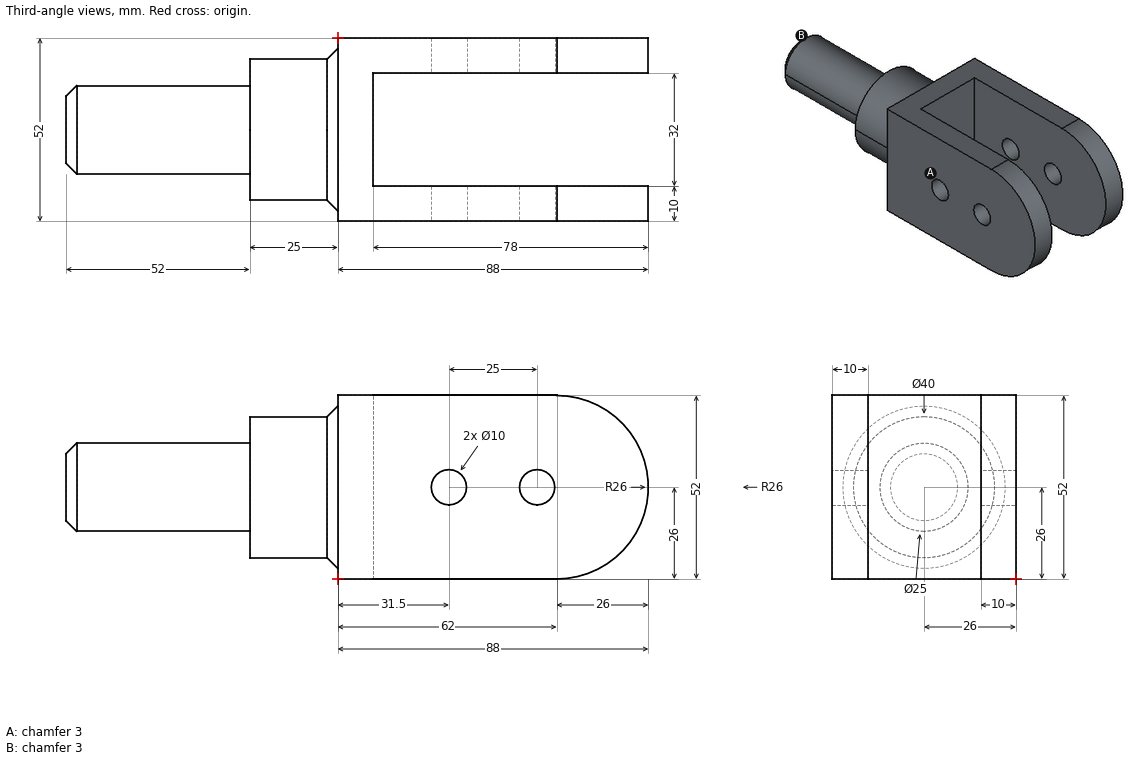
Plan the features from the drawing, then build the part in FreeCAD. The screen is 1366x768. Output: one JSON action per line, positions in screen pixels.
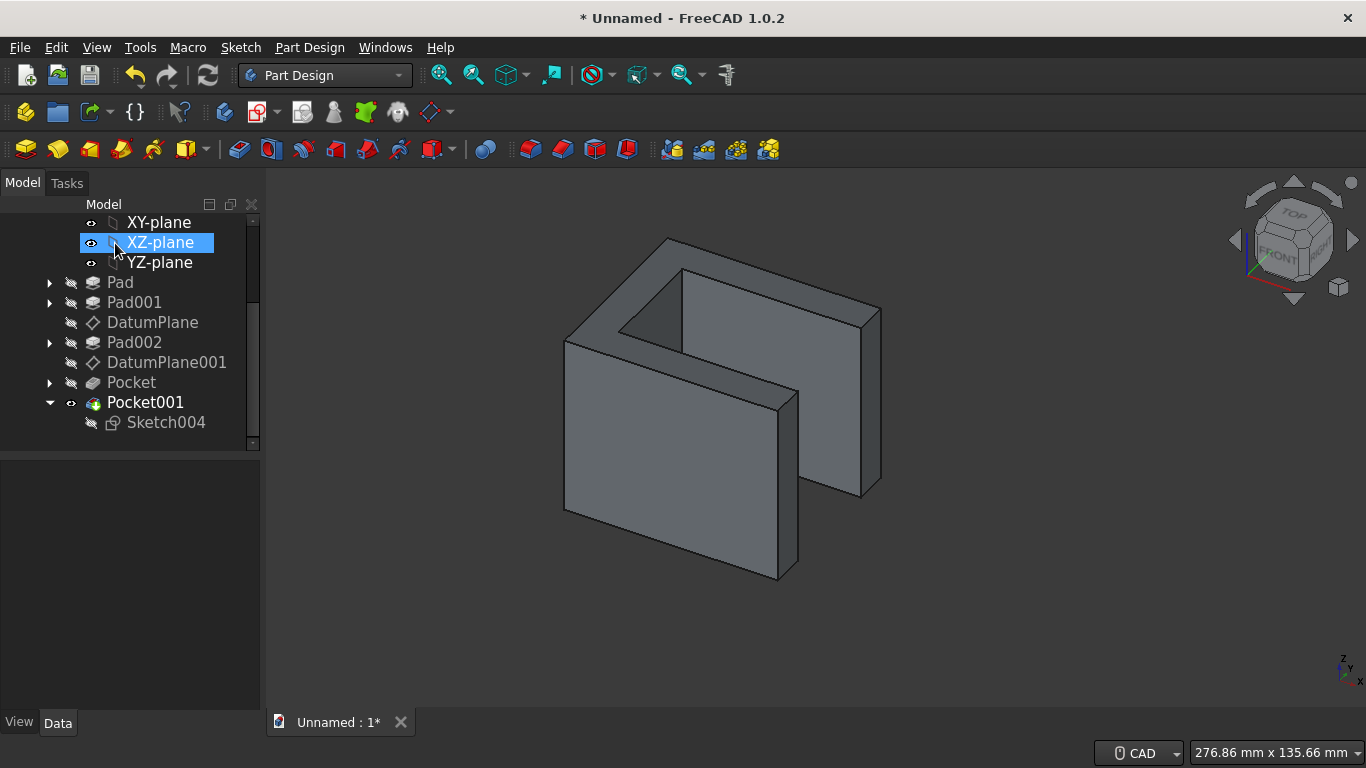
{"action": "left_click", "coordinate": [671, 460]}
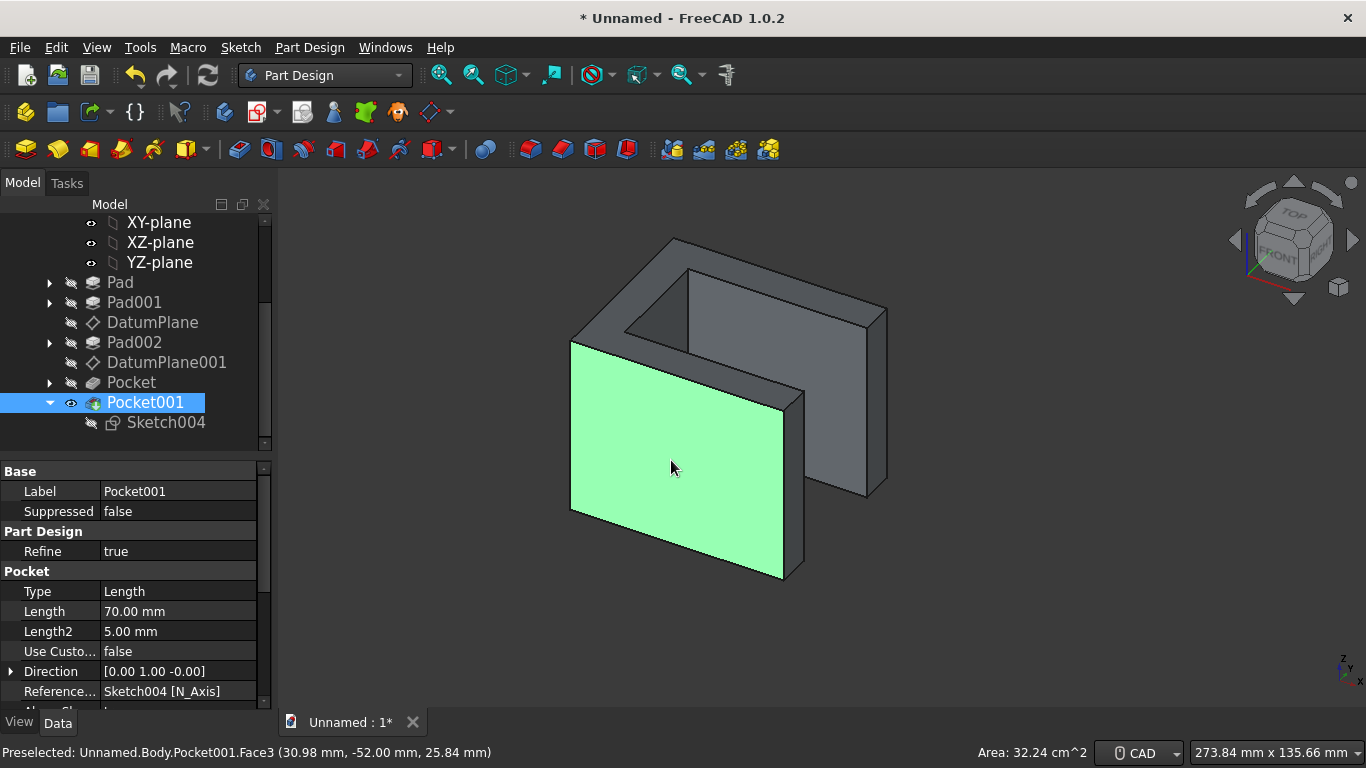
{"action": "left_click", "coordinate": [258, 112]}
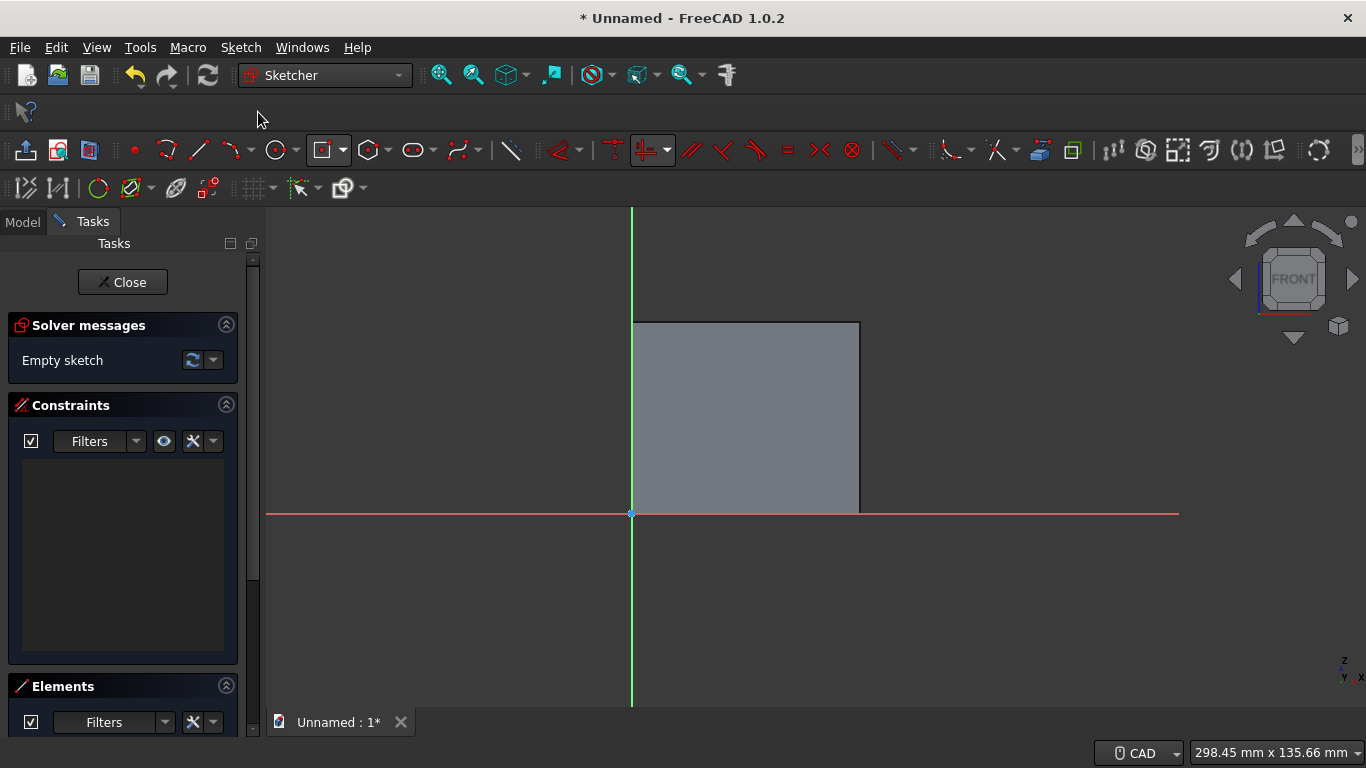
{"action": "scroll", "coordinate": [889, 338], "scroll_direction": "up", "scroll_amount": 2}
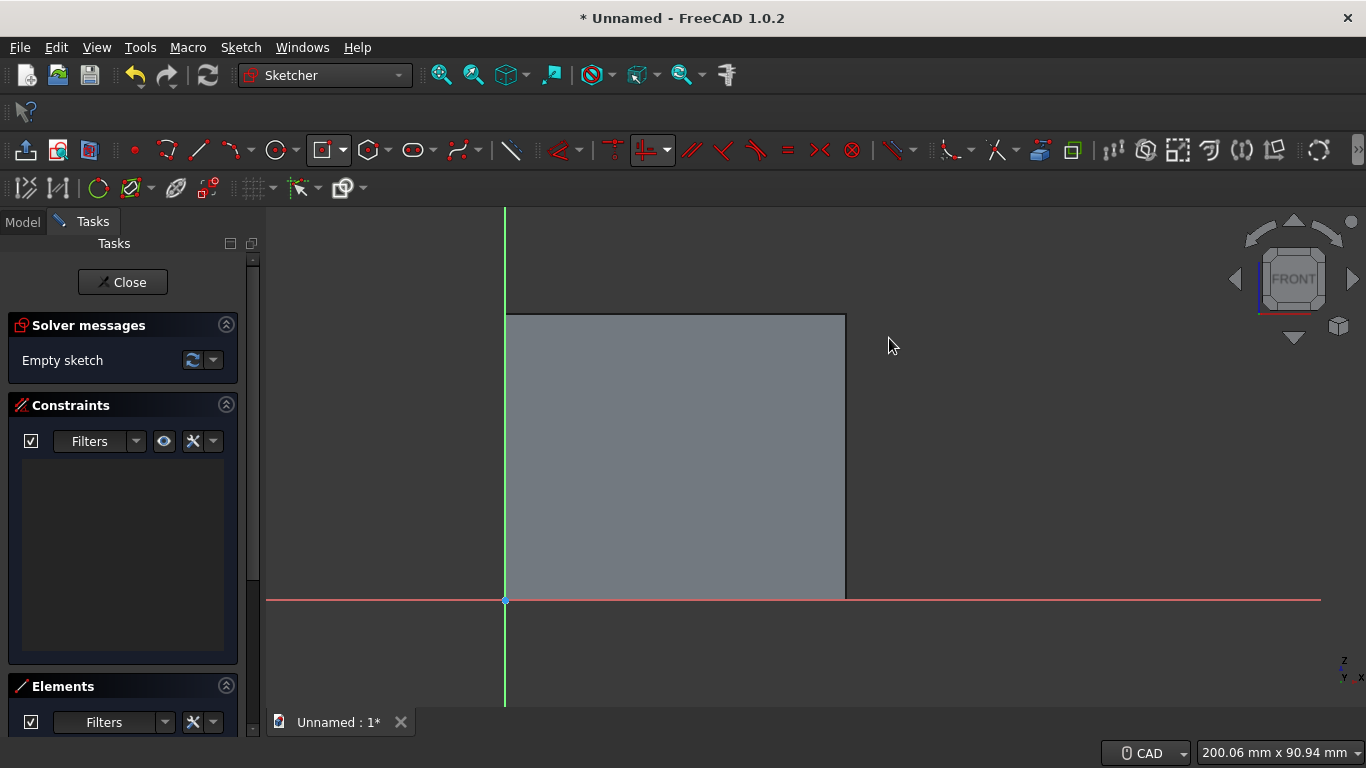
{"action": "left_click", "coordinate": [200, 150]}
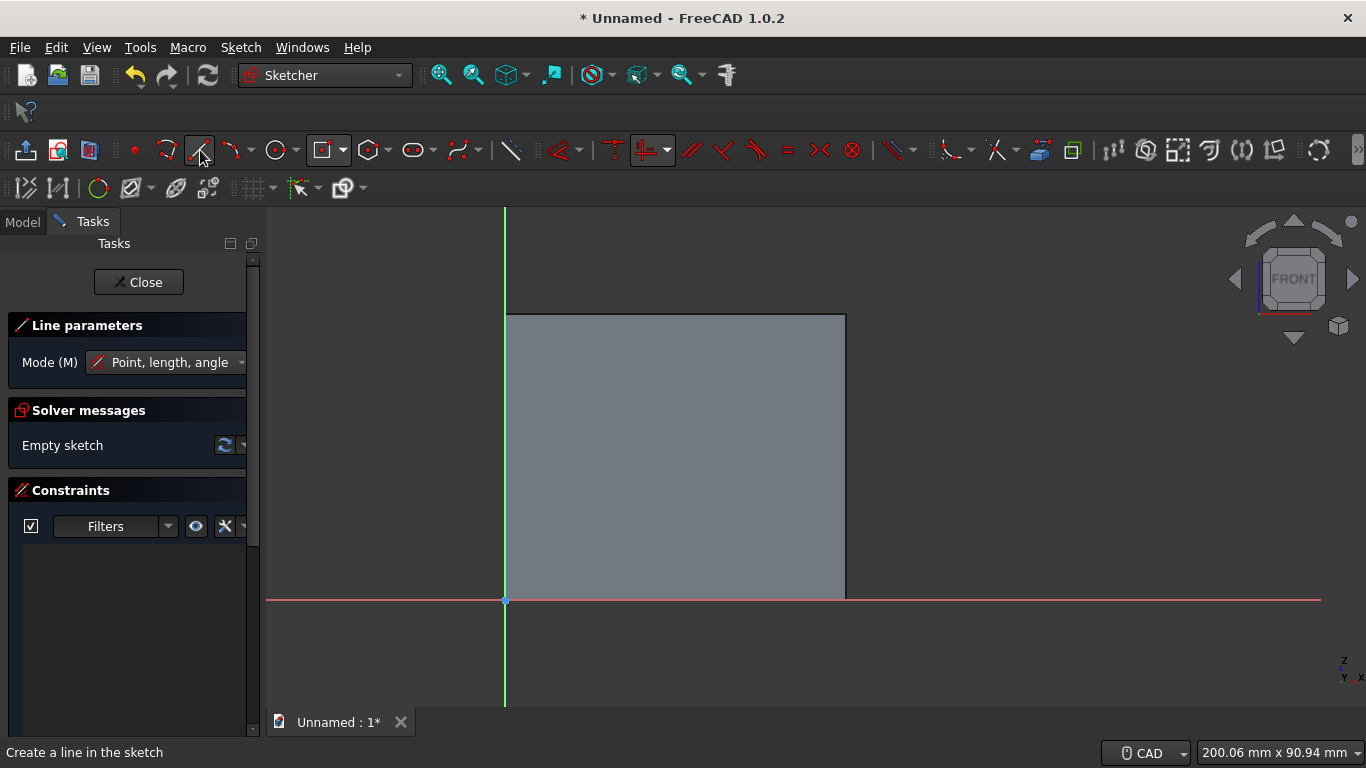
{"action": "left_click", "coordinate": [846, 314]}
{"action": "left_click", "coordinate": [846, 600]}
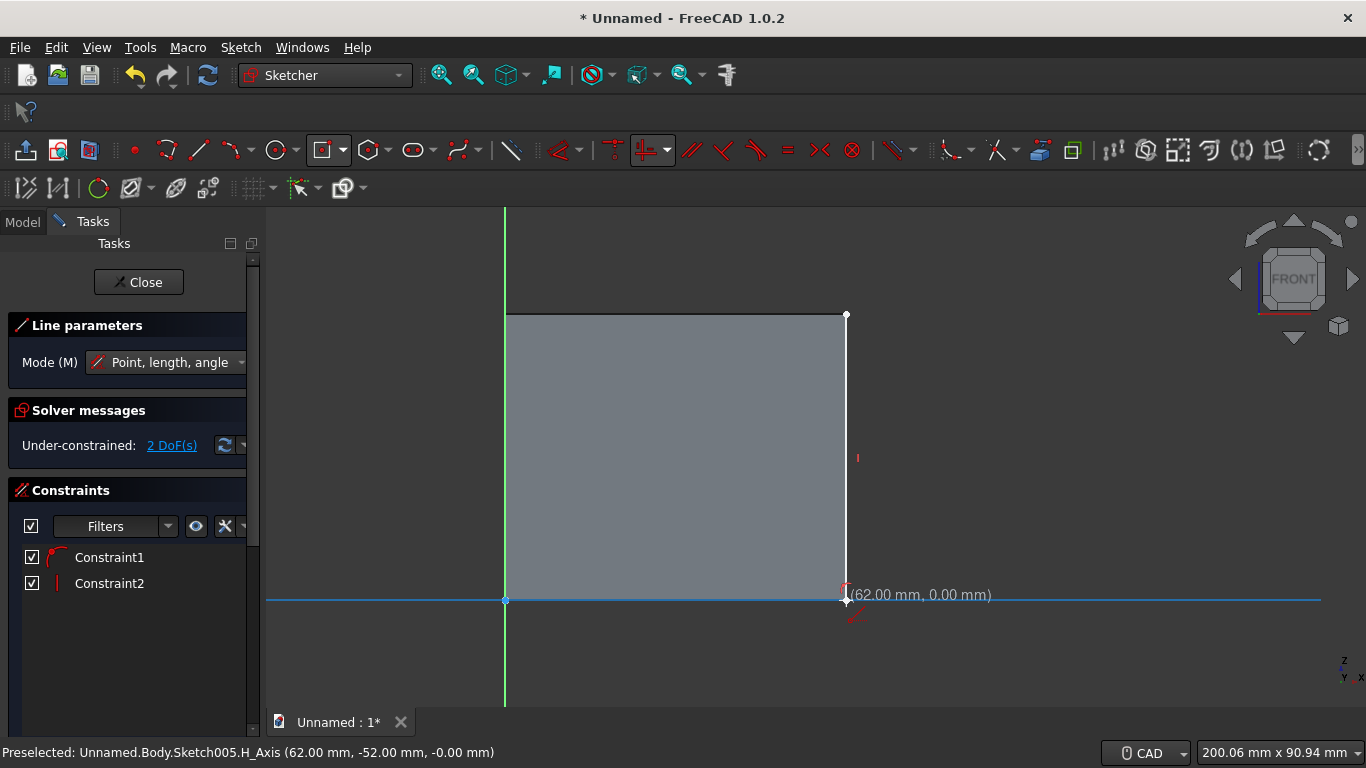
{"action": "left_click", "coordinate": [232, 150]}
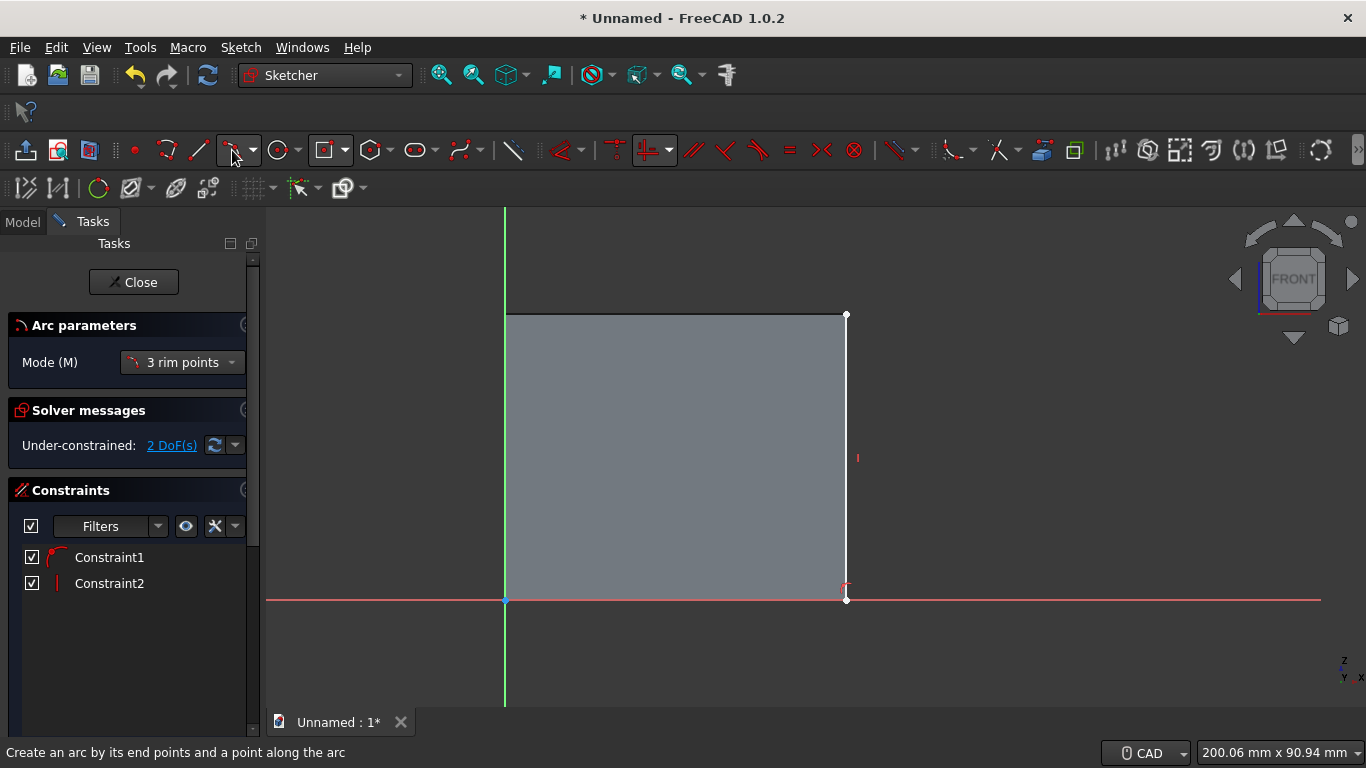
{"action": "left_click", "coordinate": [846, 600]}
{"action": "left_click", "coordinate": [846, 315]}
{"action": "left_click", "coordinate": [989, 457]}
{"action": "key", "text": "Escape"}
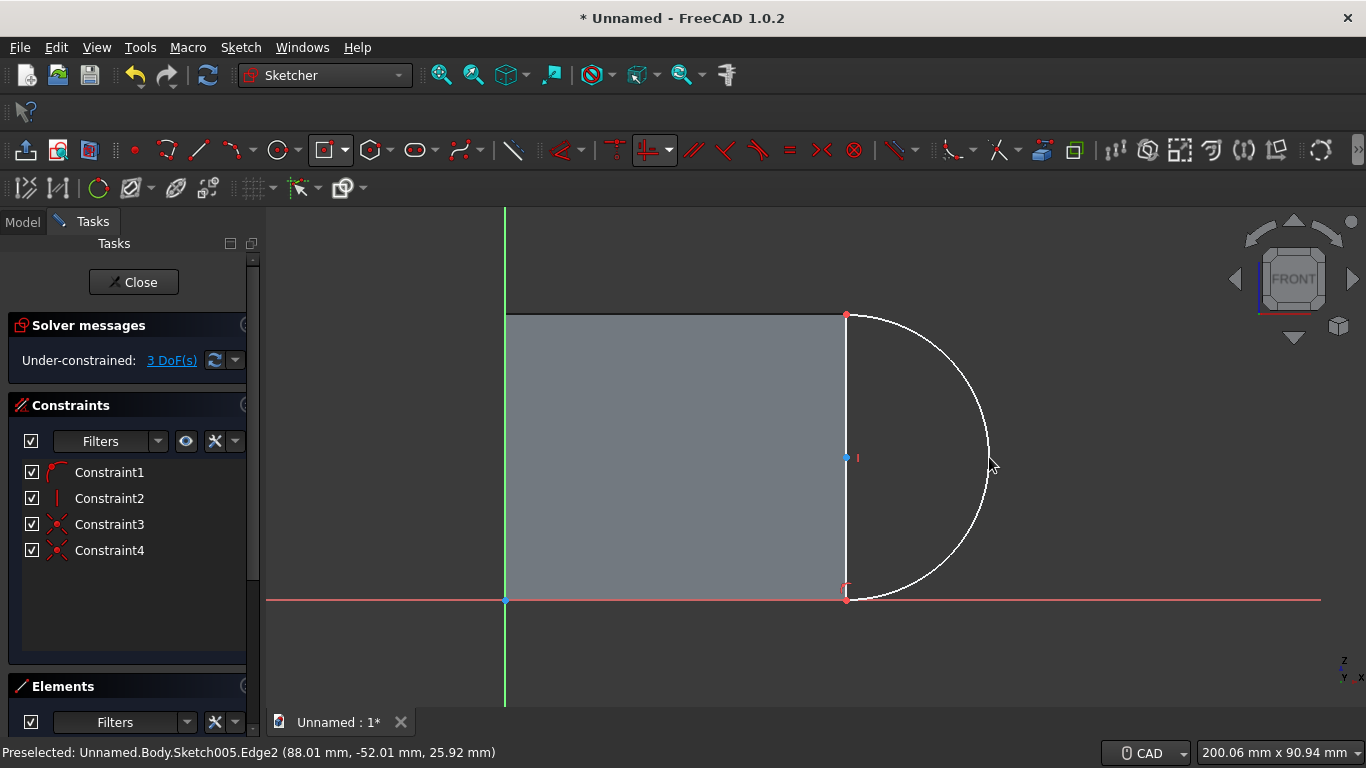
{"action": "left_click", "coordinate": [560, 150]}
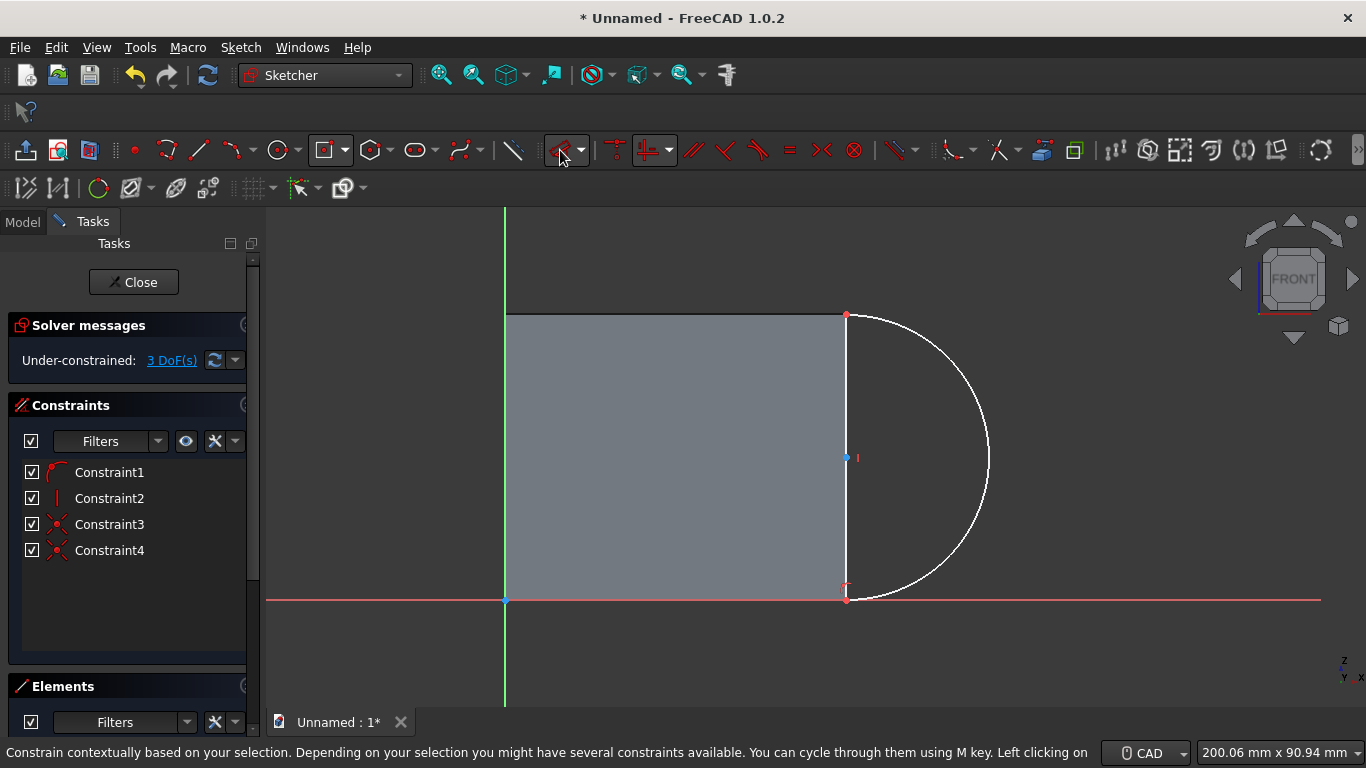
{"action": "left_click", "coordinate": [962, 541]}
{"action": "left_click", "coordinate": [988, 560]}